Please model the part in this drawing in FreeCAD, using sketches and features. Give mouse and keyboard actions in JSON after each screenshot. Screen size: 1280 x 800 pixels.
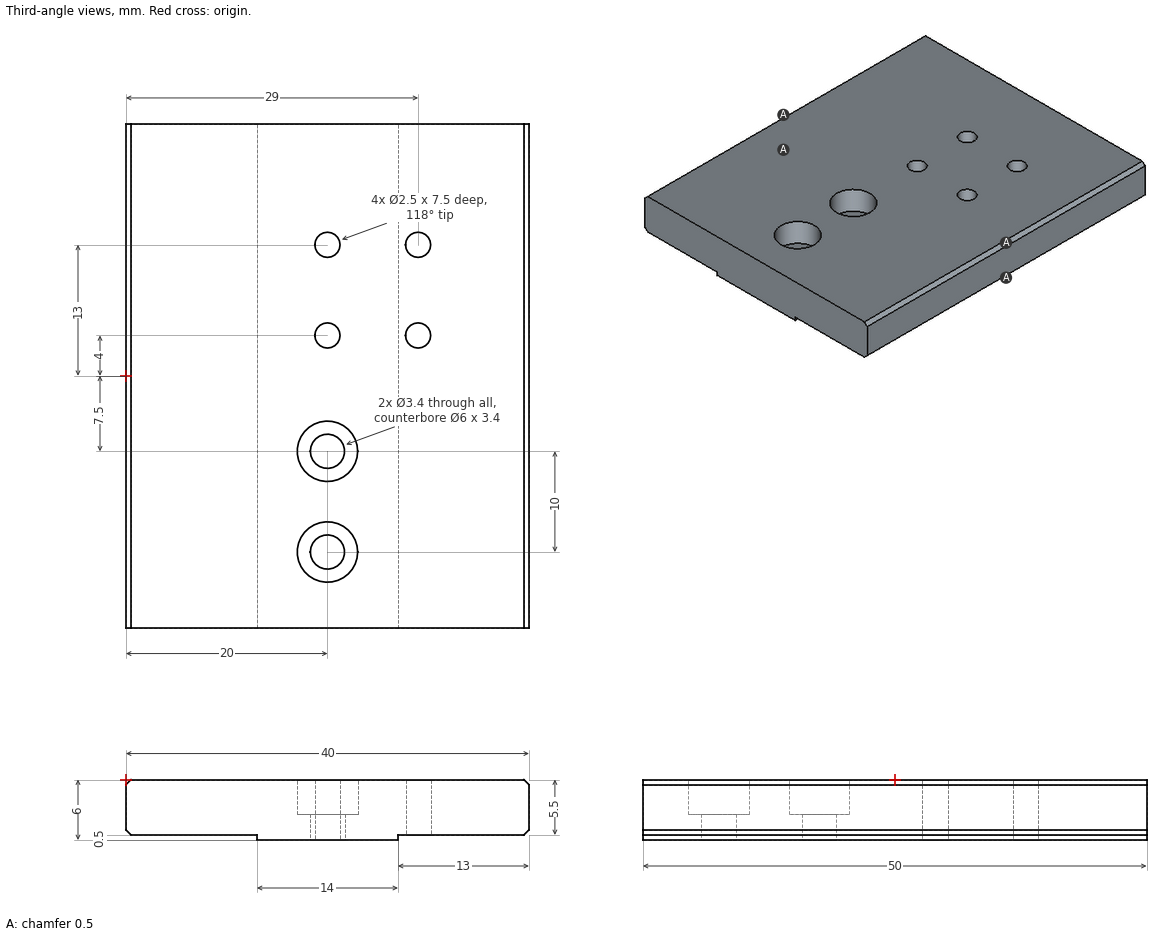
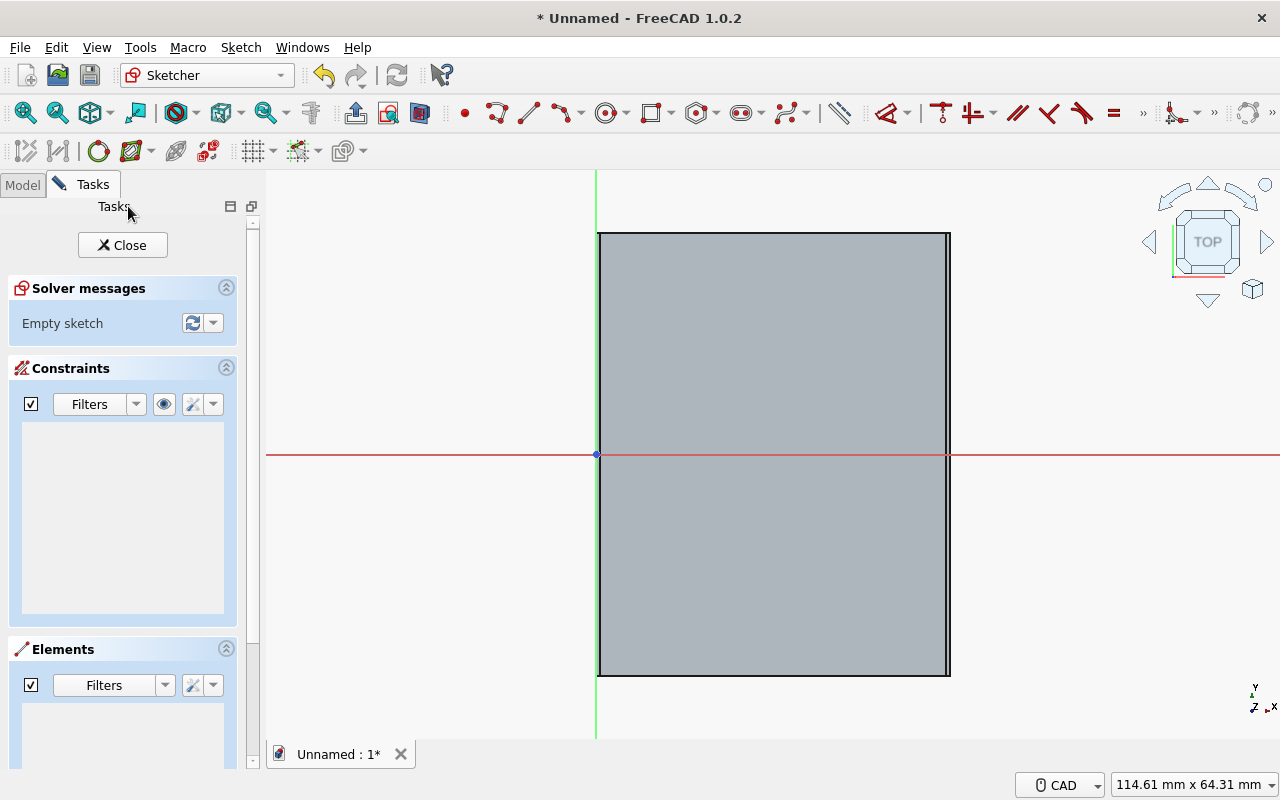
{"action": "scroll", "coordinate": [682, 609], "scroll_direction": "up", "scroll_amount": 4}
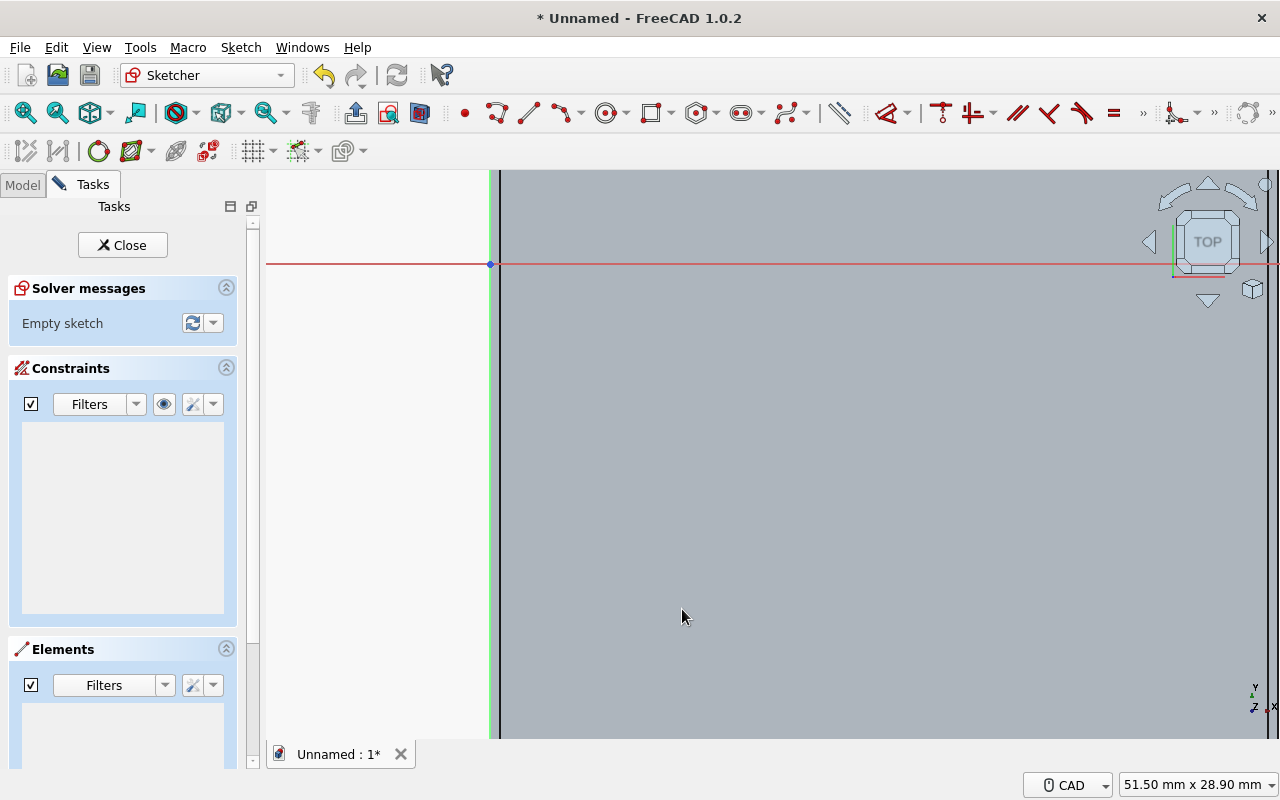
{"action": "left_click", "coordinate": [606, 114]}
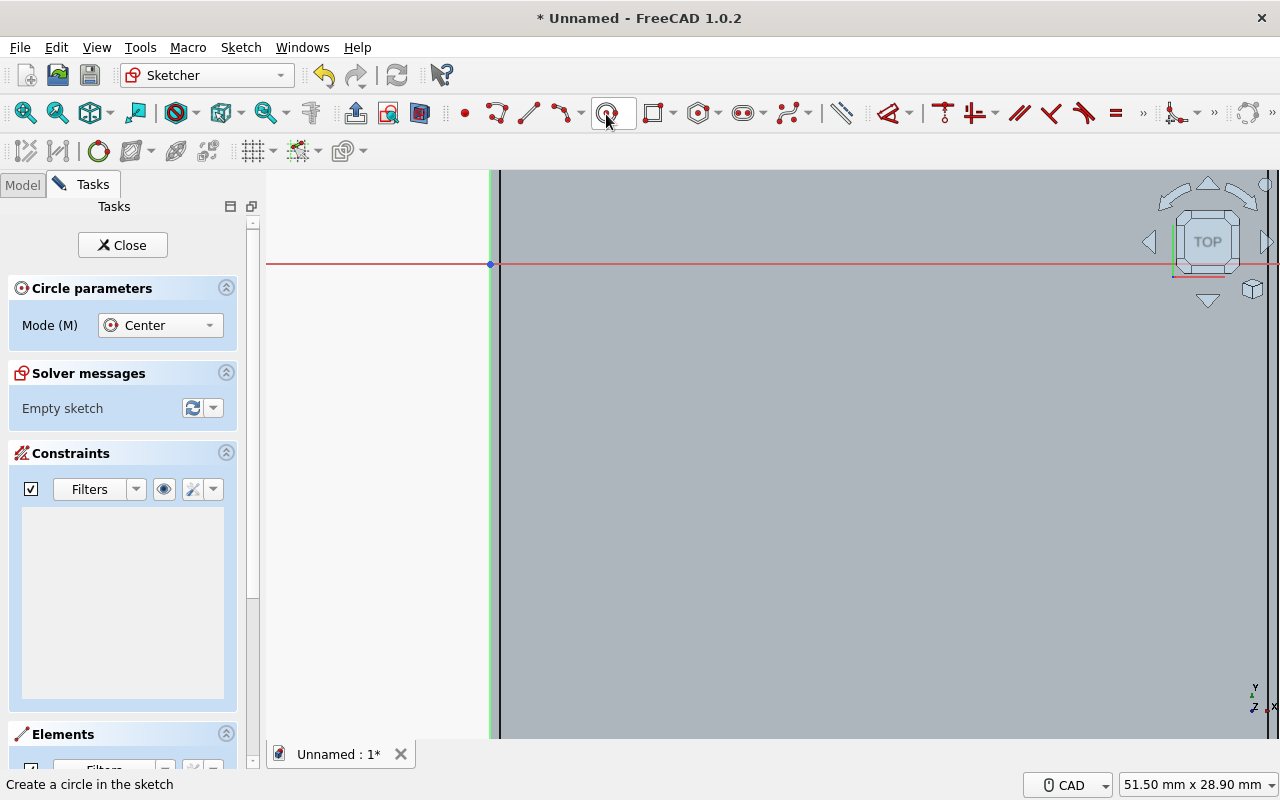
{"action": "left_click", "coordinate": [884, 412]}
{"action": "mouse_move", "coordinate": [908, 388]}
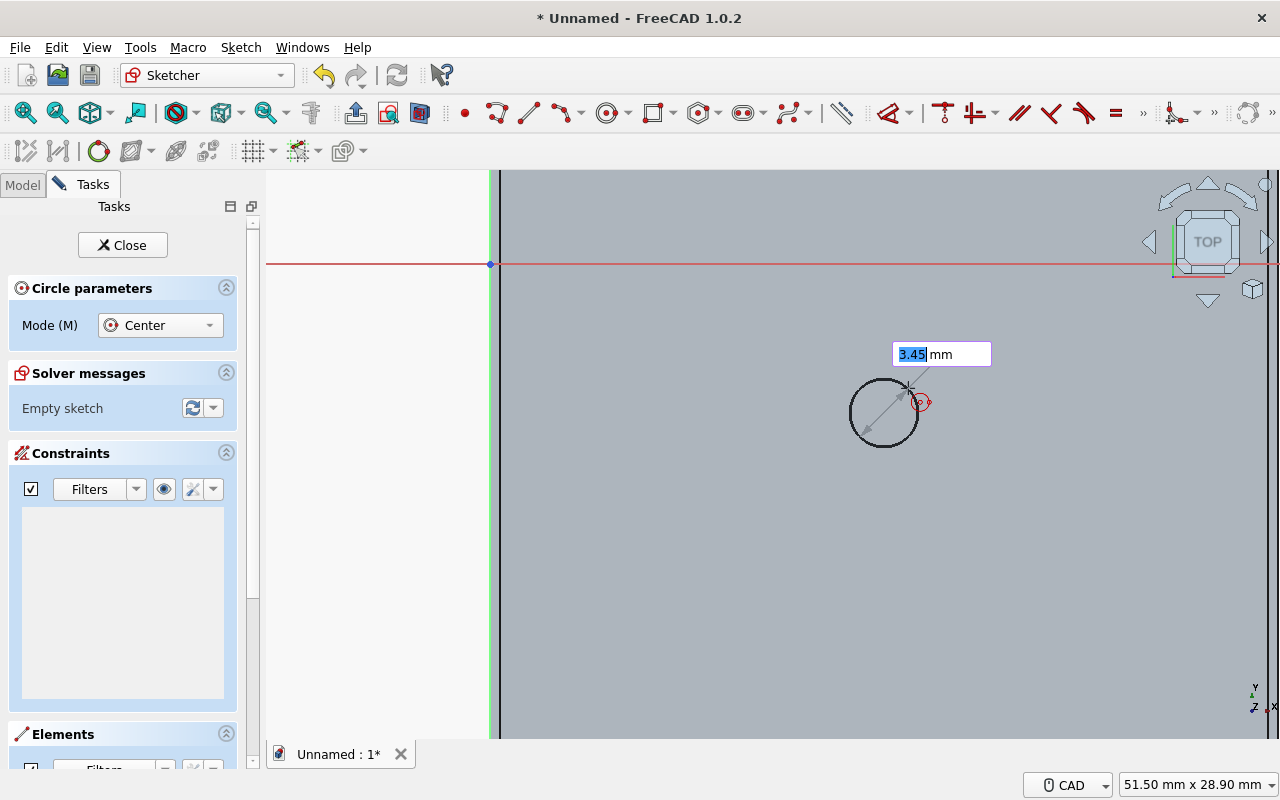
{"action": "type", "text": "3.4"}
{"action": "key", "text": "Return"}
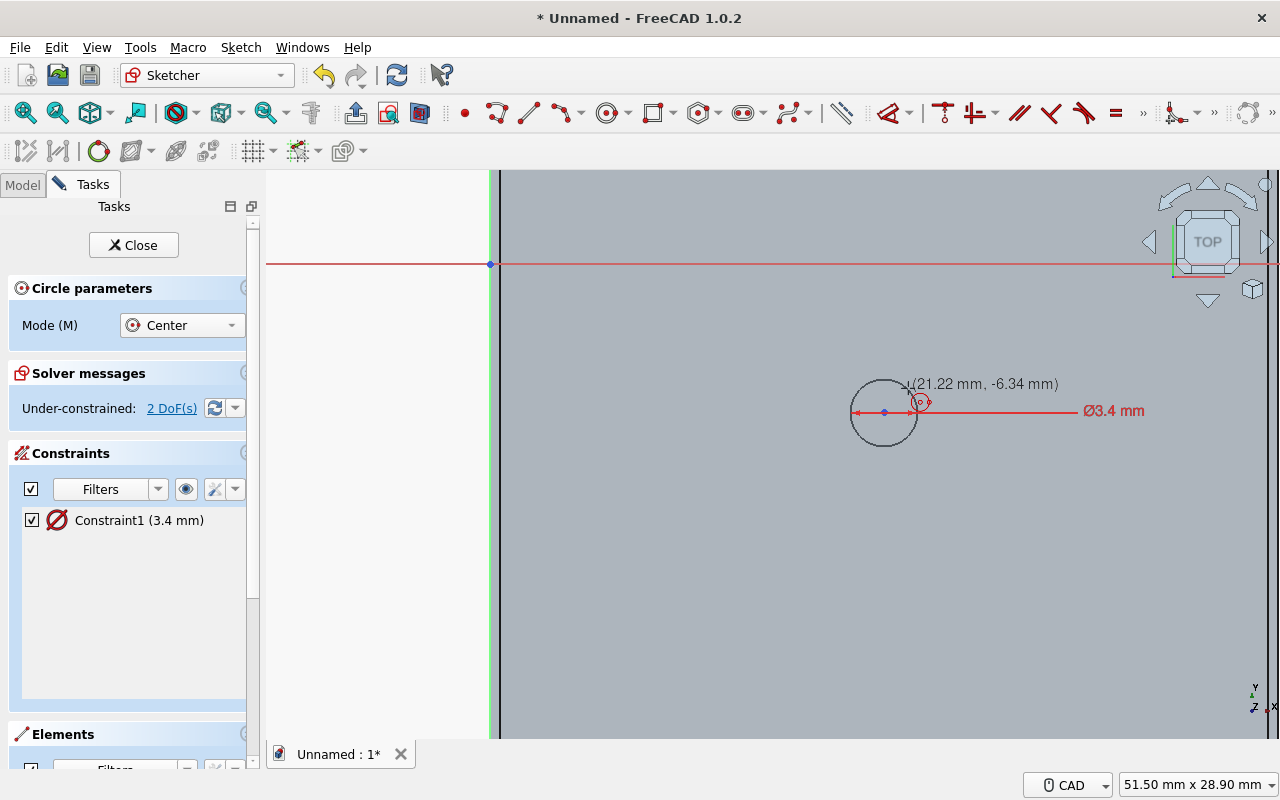
{"action": "left_click", "coordinate": [884, 609]}
{"action": "mouse_move", "coordinate": [908, 585]}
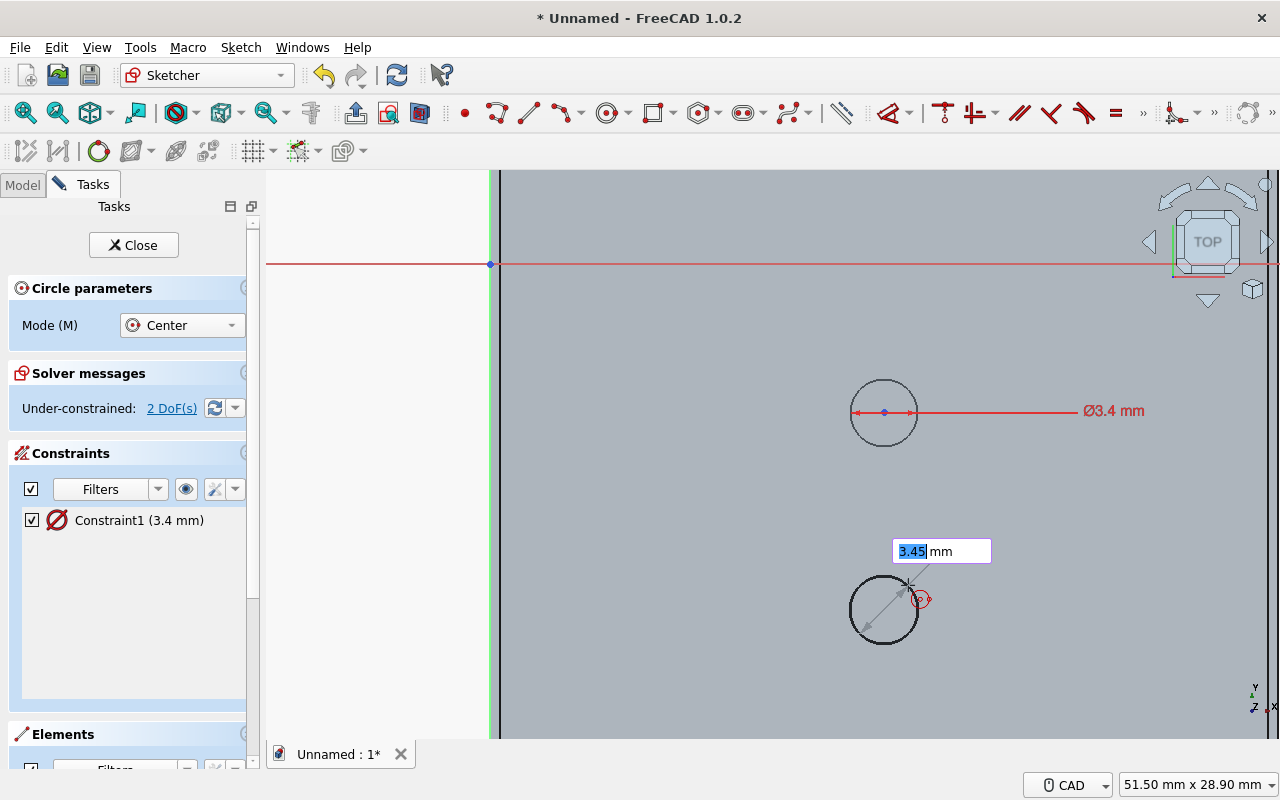
{"action": "type", "text": "3.4"}
{"action": "key", "text": "Return"}
{"action": "key", "text": "Escape"}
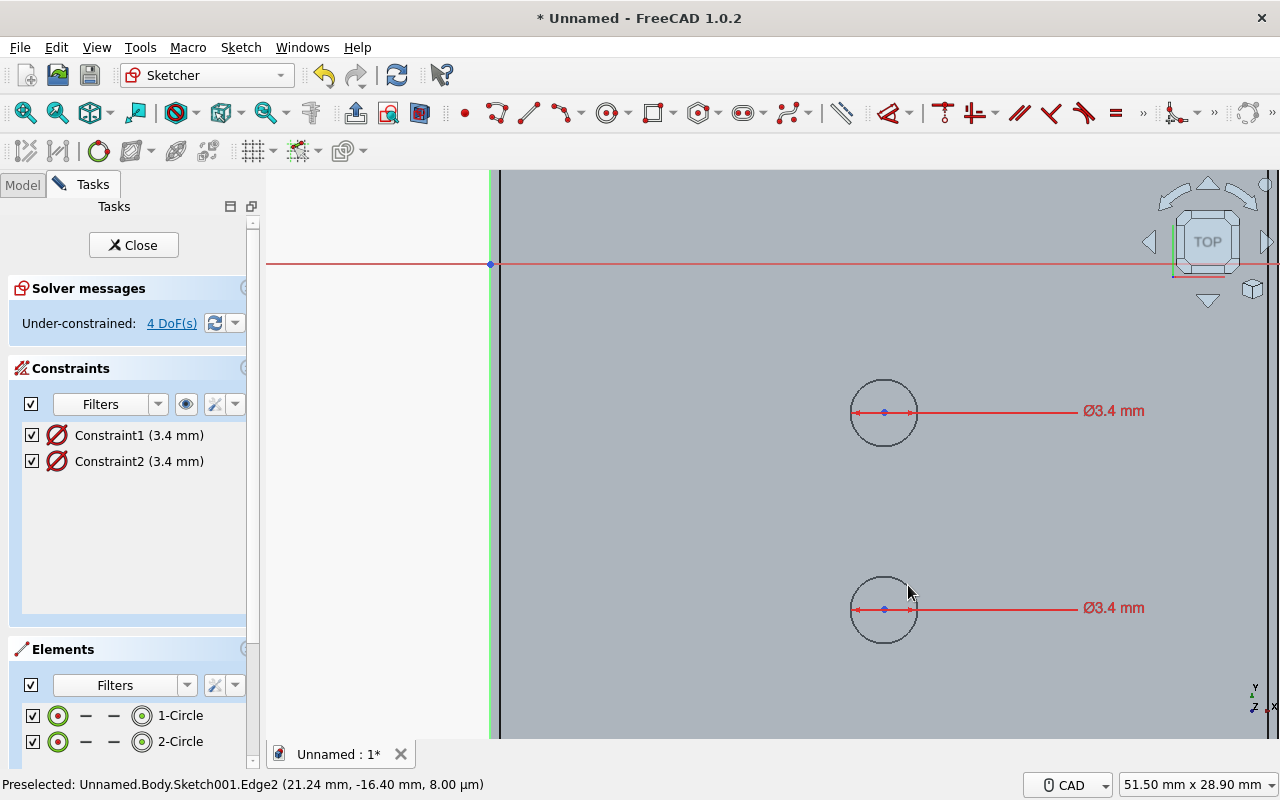
{"action": "left_click", "coordinate": [888, 114]}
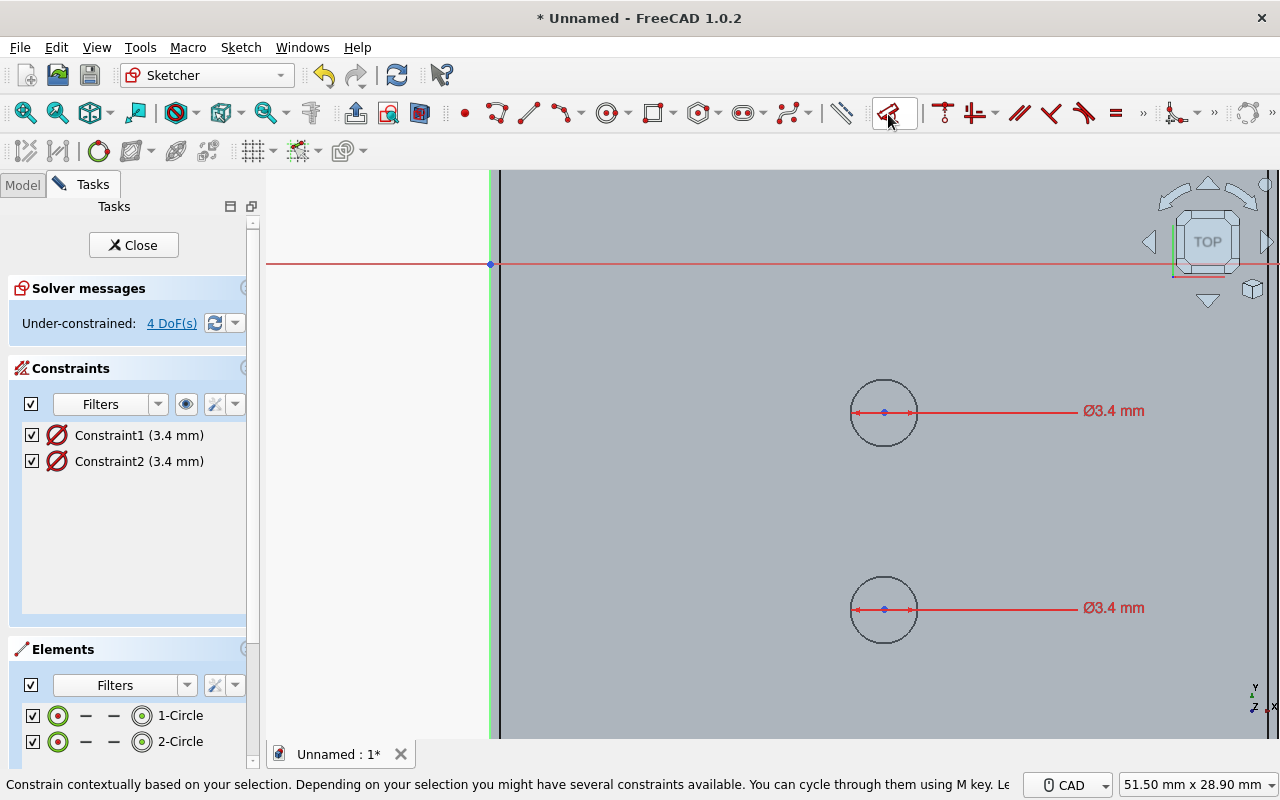
{"action": "left_click", "coordinate": [884, 413]}
{"action": "left_click", "coordinate": [687, 230]}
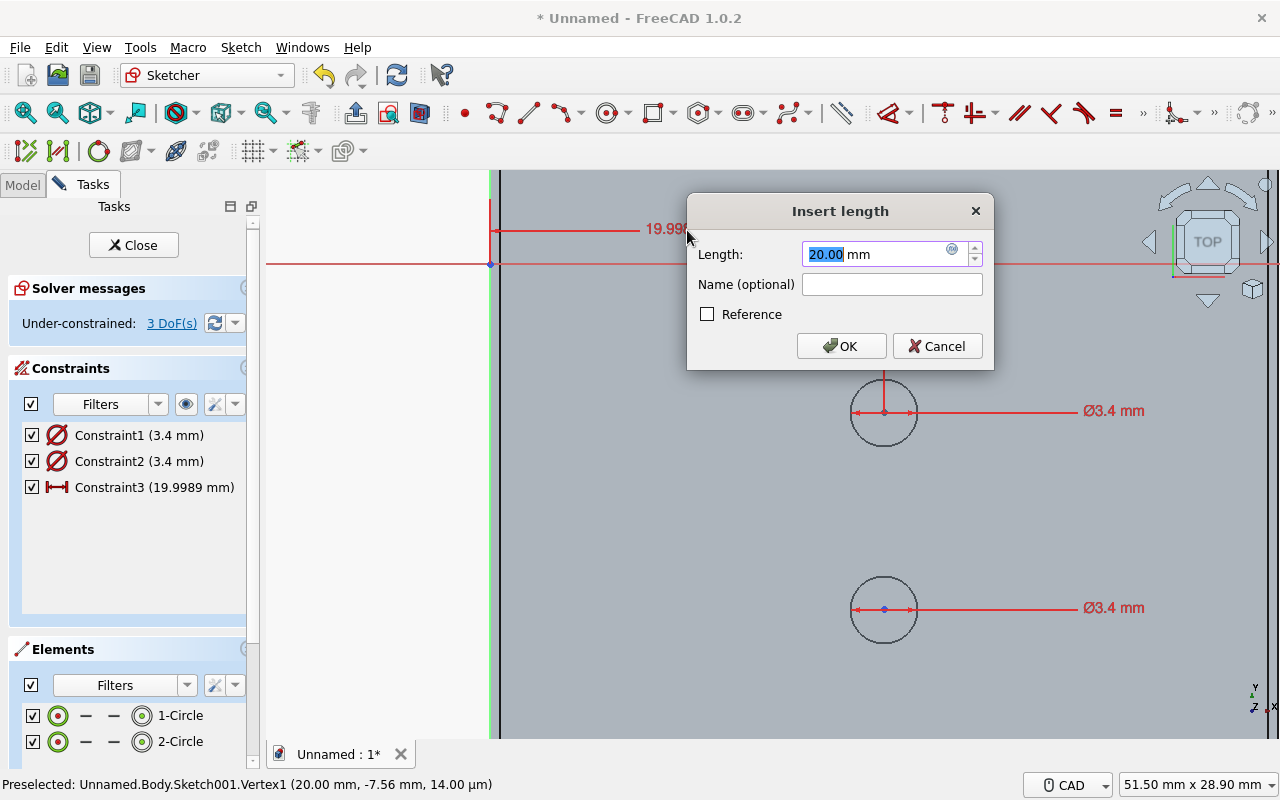
{"action": "type", "text": "20"}
{"action": "key", "text": "Return"}